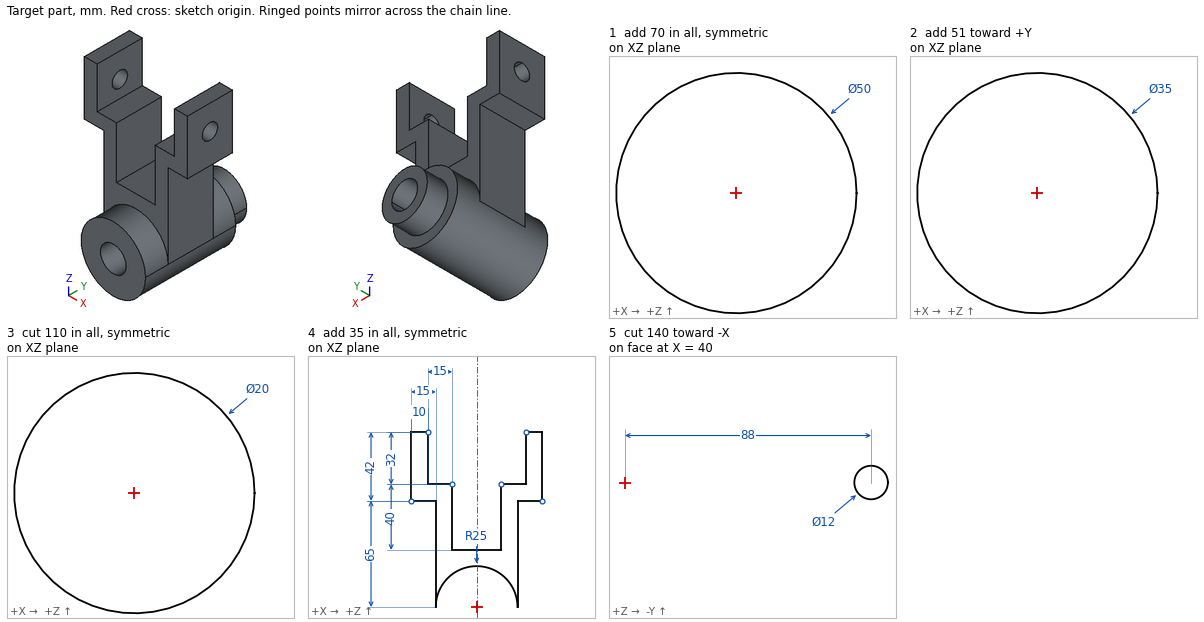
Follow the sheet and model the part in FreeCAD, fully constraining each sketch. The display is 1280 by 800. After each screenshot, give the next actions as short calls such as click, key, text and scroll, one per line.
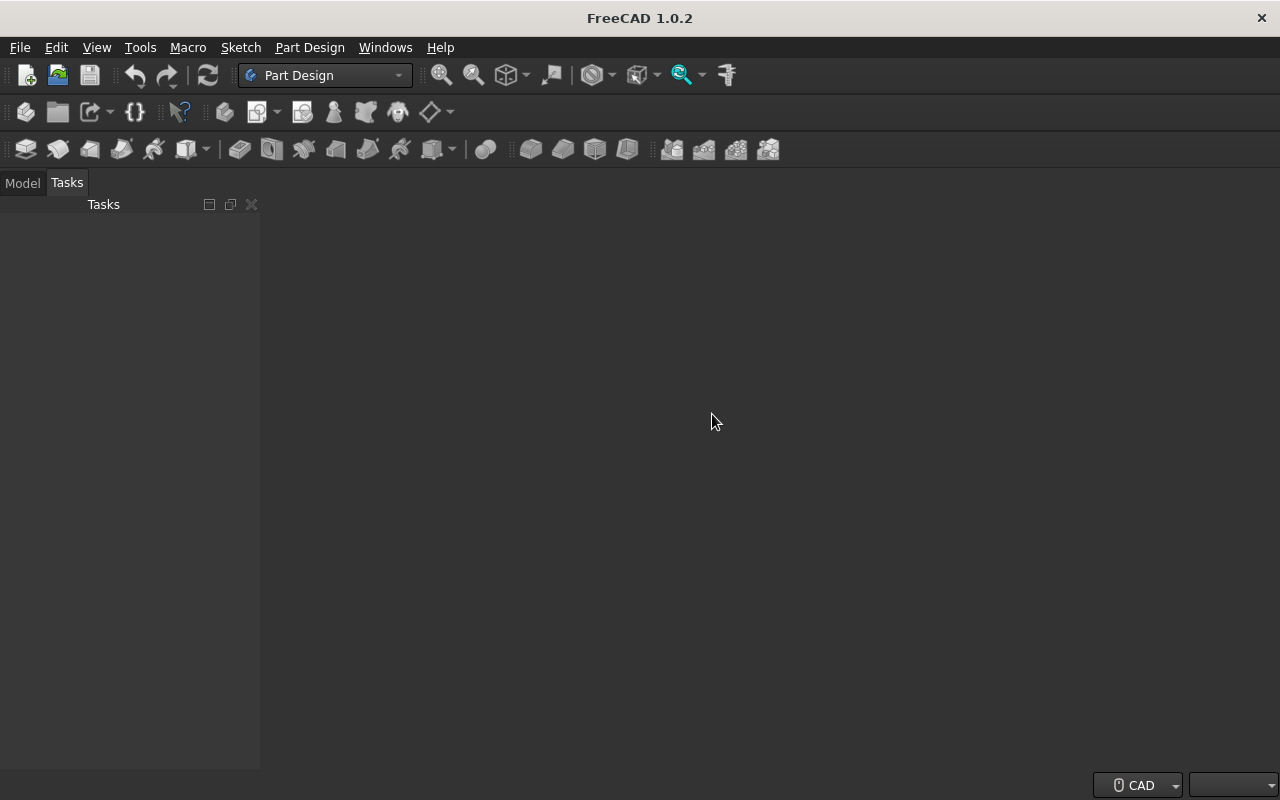
click(26, 76)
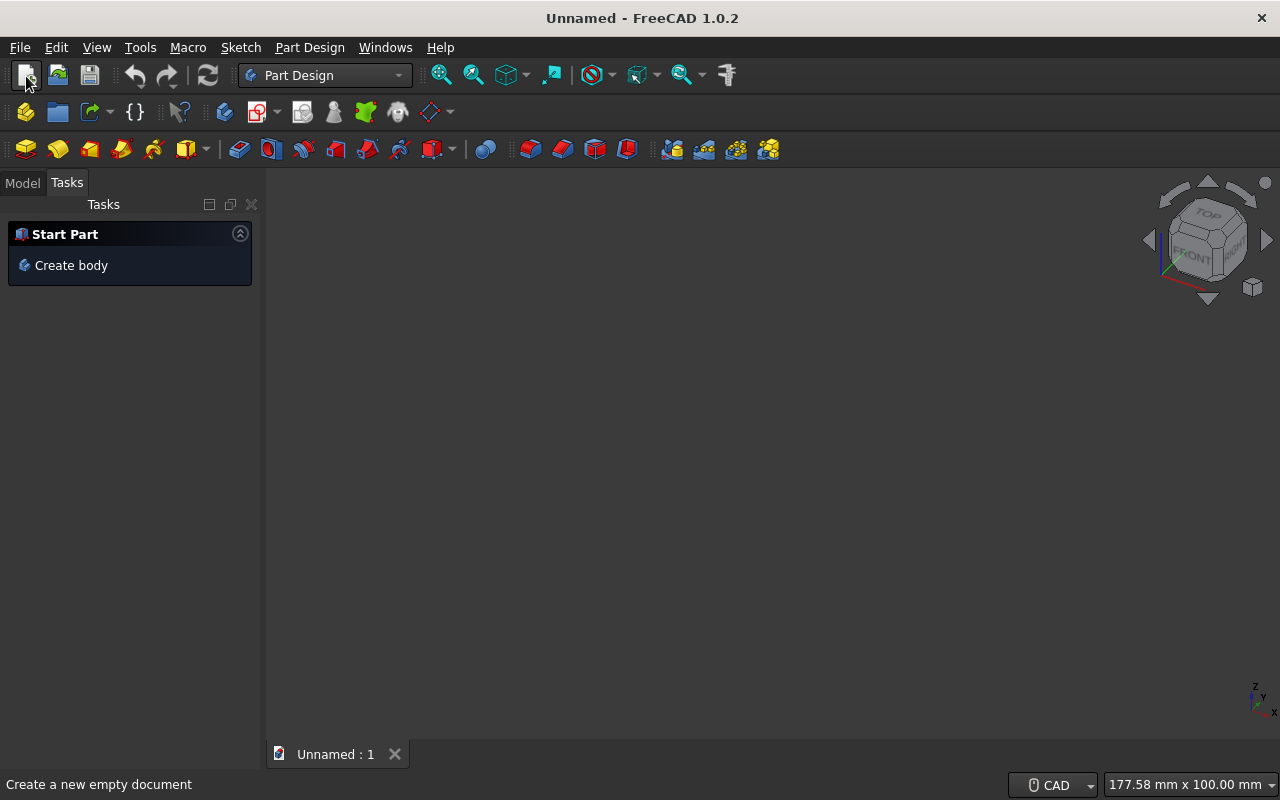
click(258, 112)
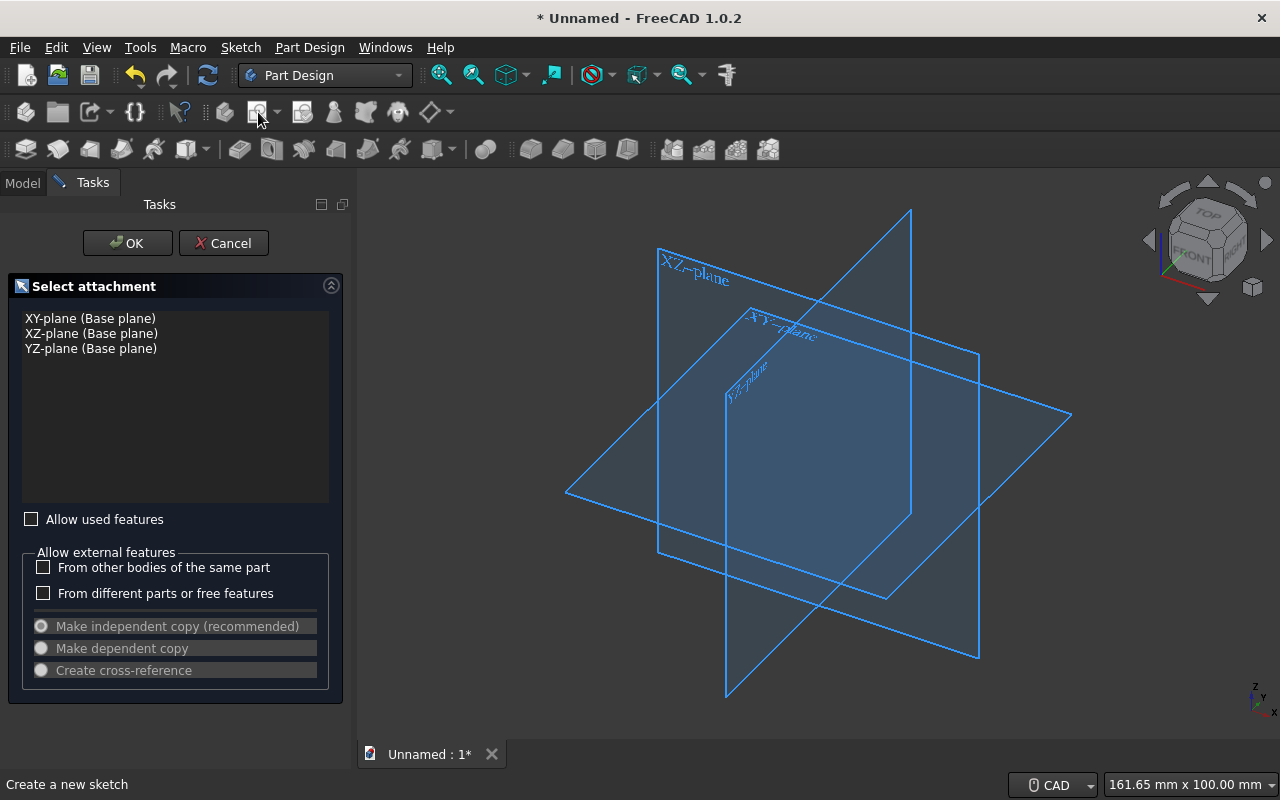
click(82, 334)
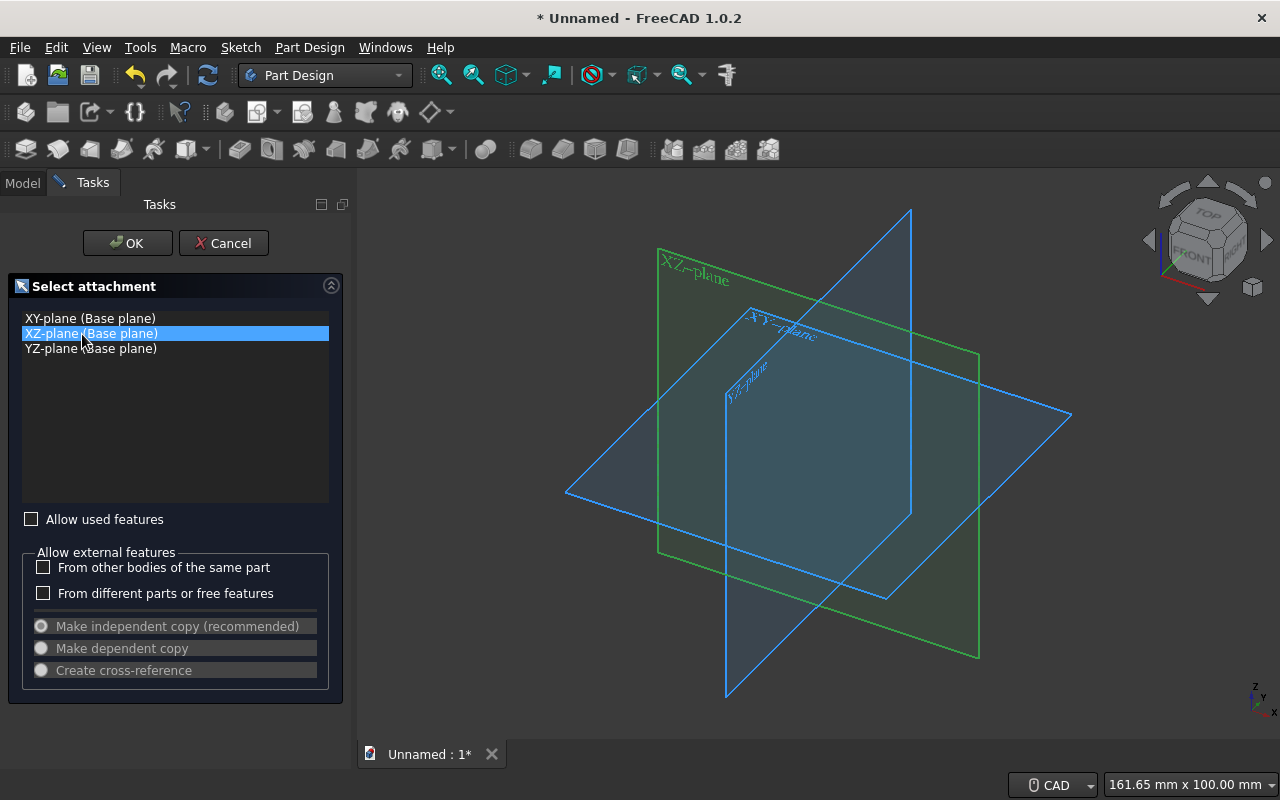
click(128, 243)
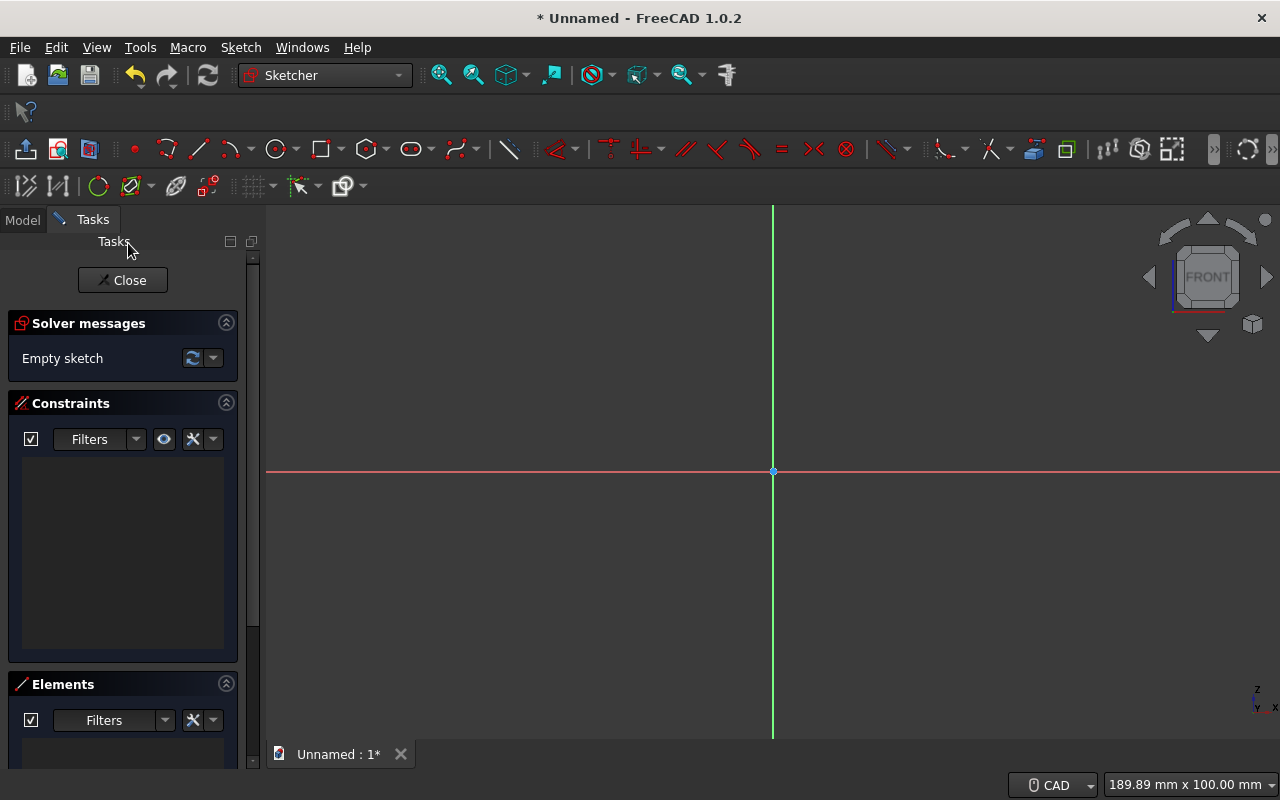
click(276, 150)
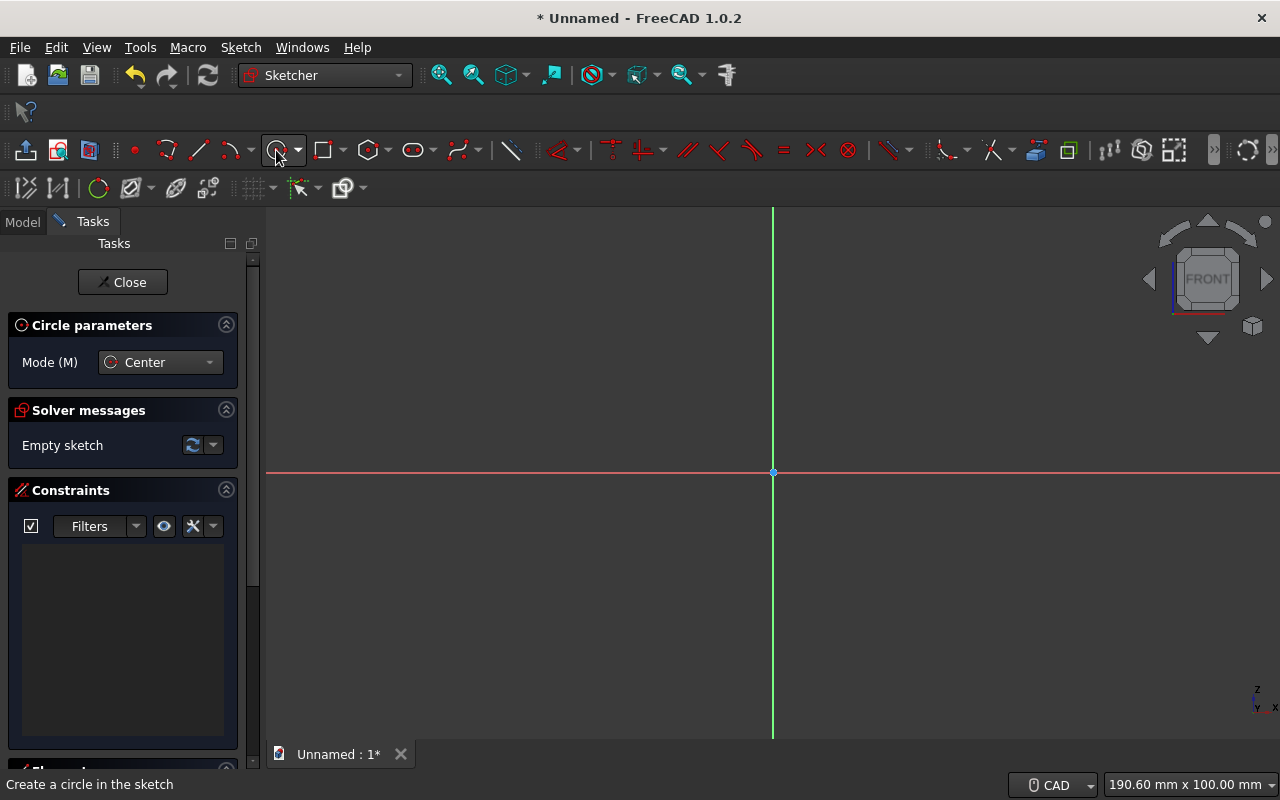
click(773, 473)
click(867, 379)
key(Escape)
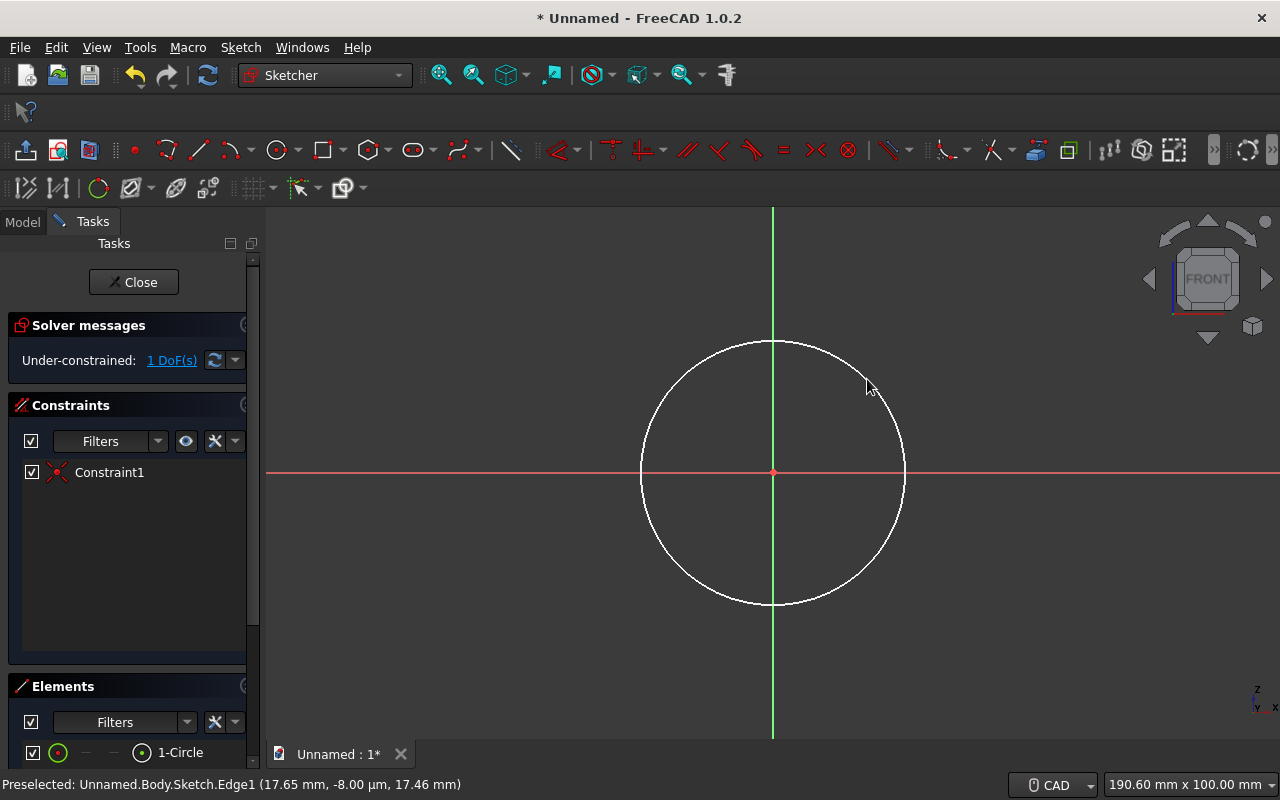
click(558, 150)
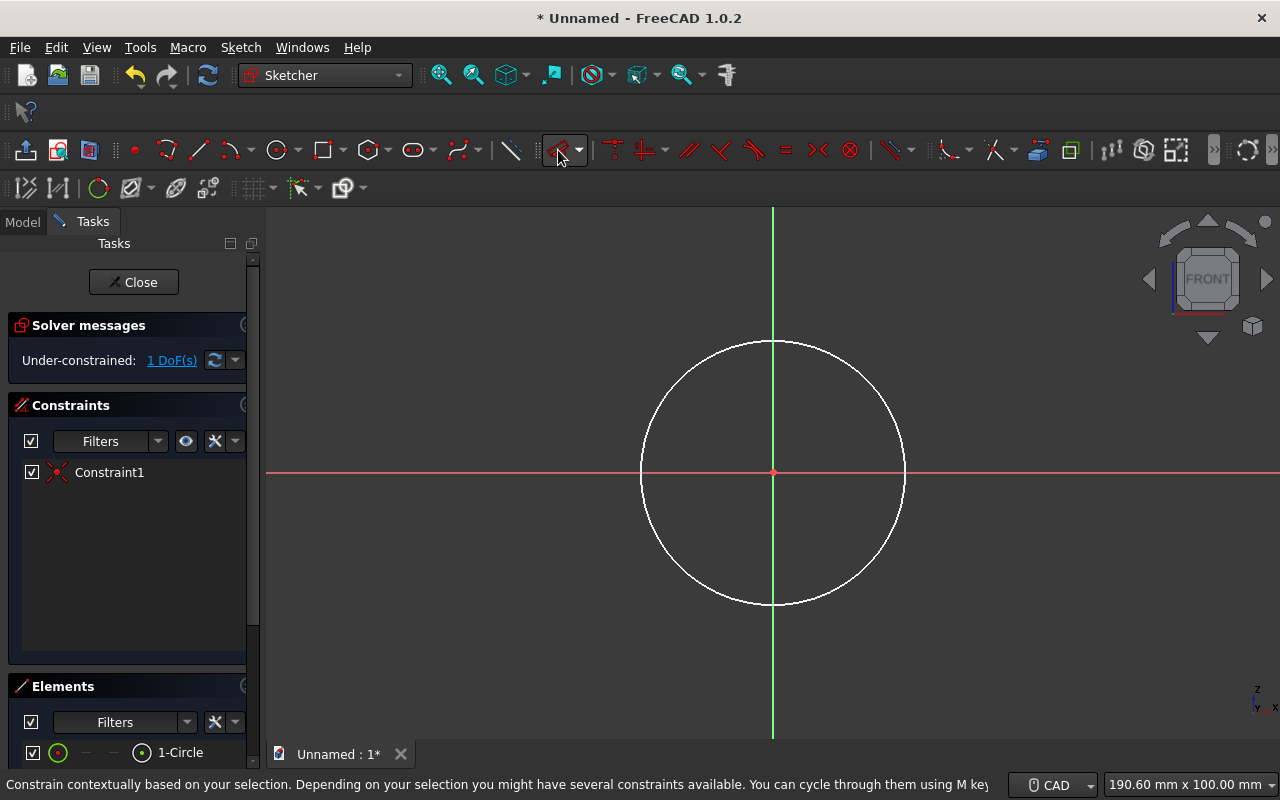
click(866, 379)
click(889, 356)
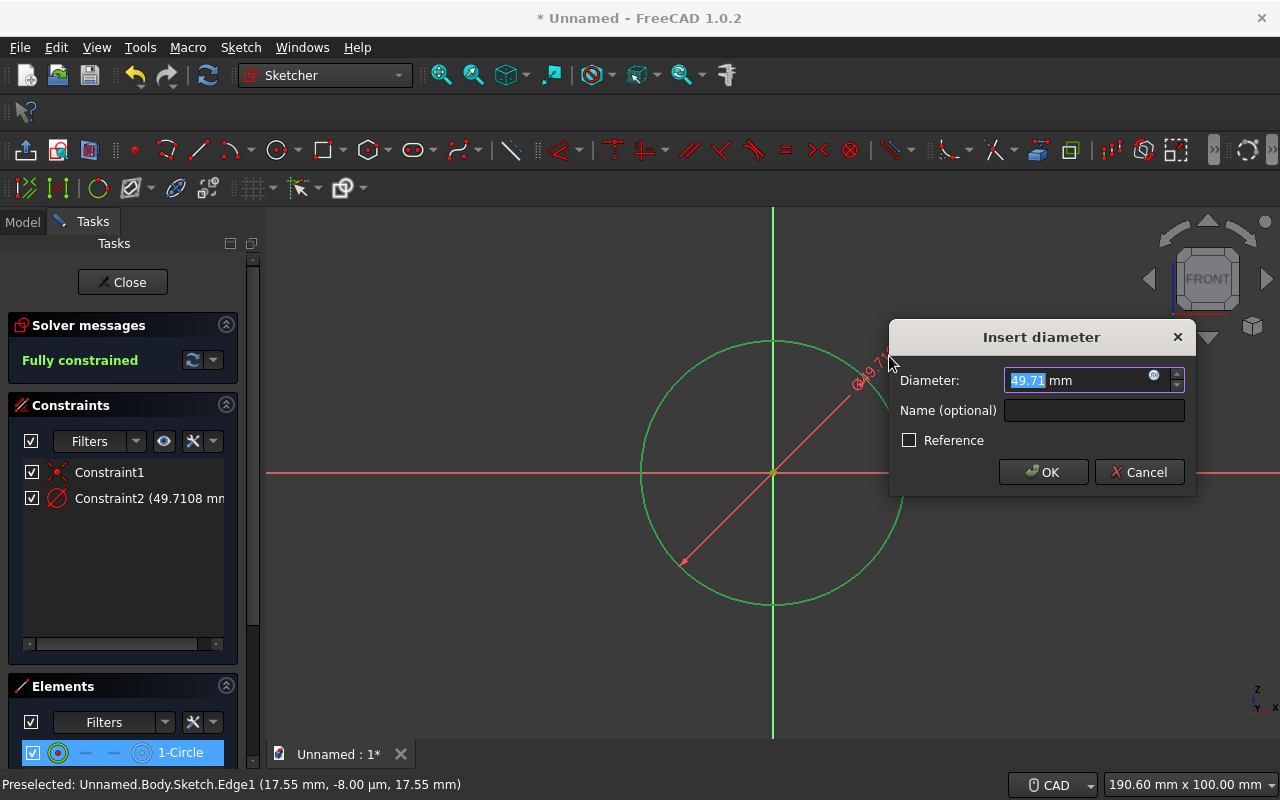
text(50)
key(Return)
key(Escape)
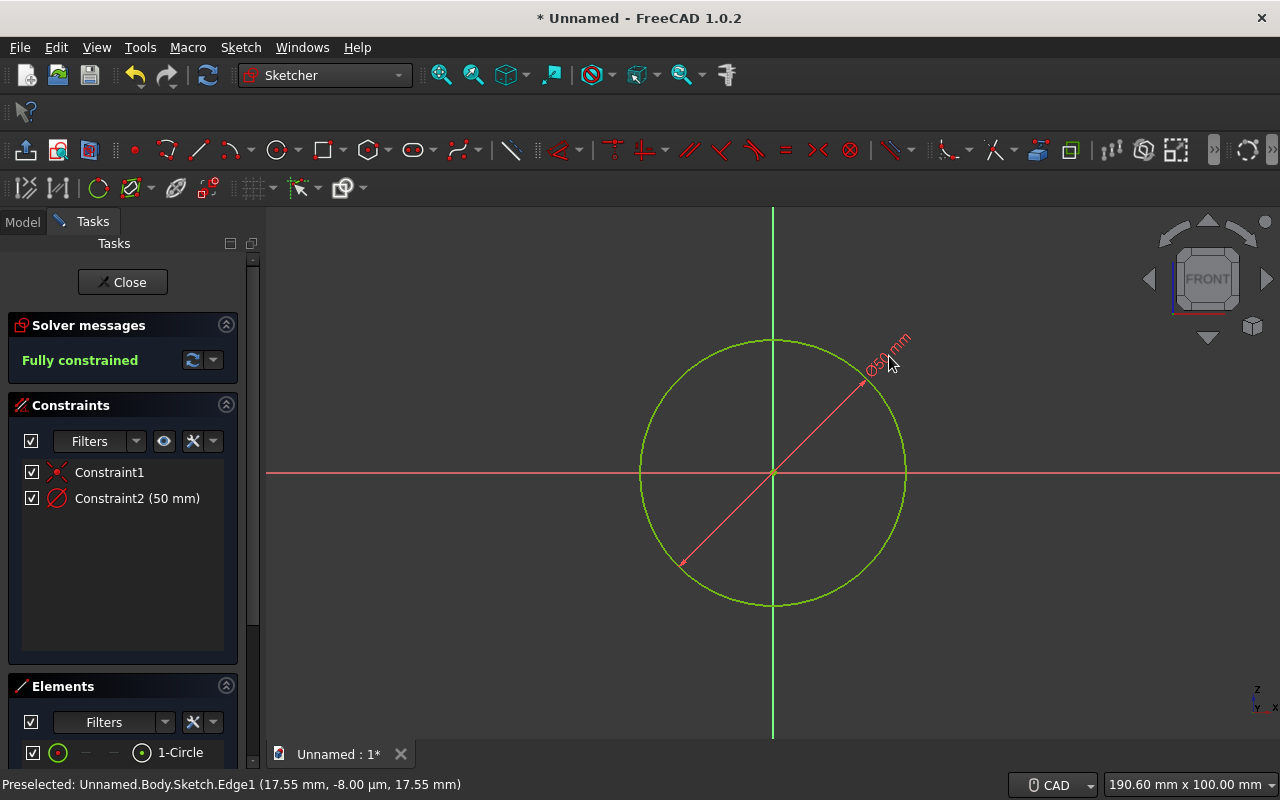
click(123, 282)